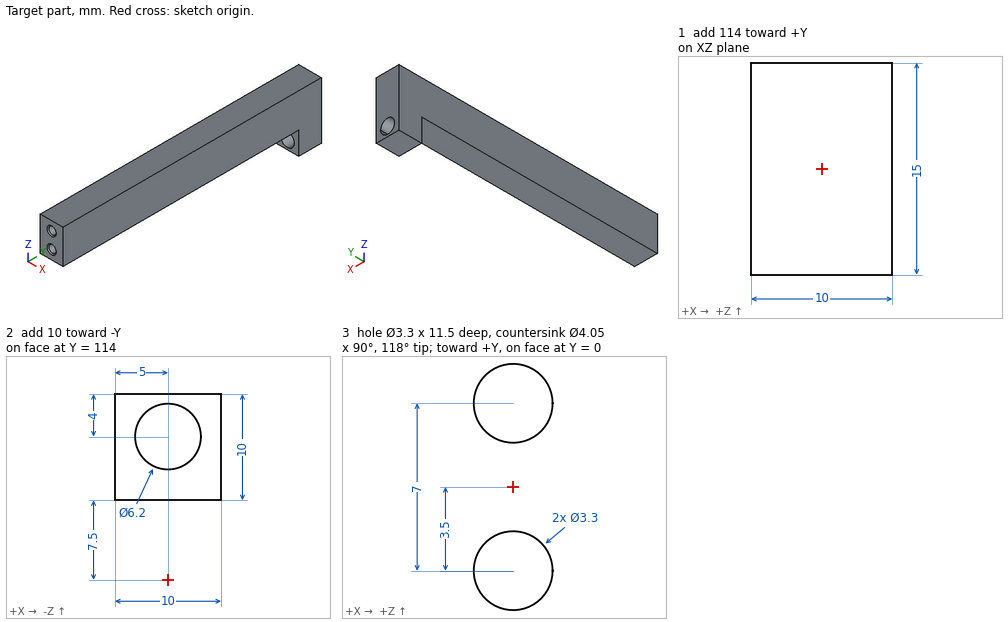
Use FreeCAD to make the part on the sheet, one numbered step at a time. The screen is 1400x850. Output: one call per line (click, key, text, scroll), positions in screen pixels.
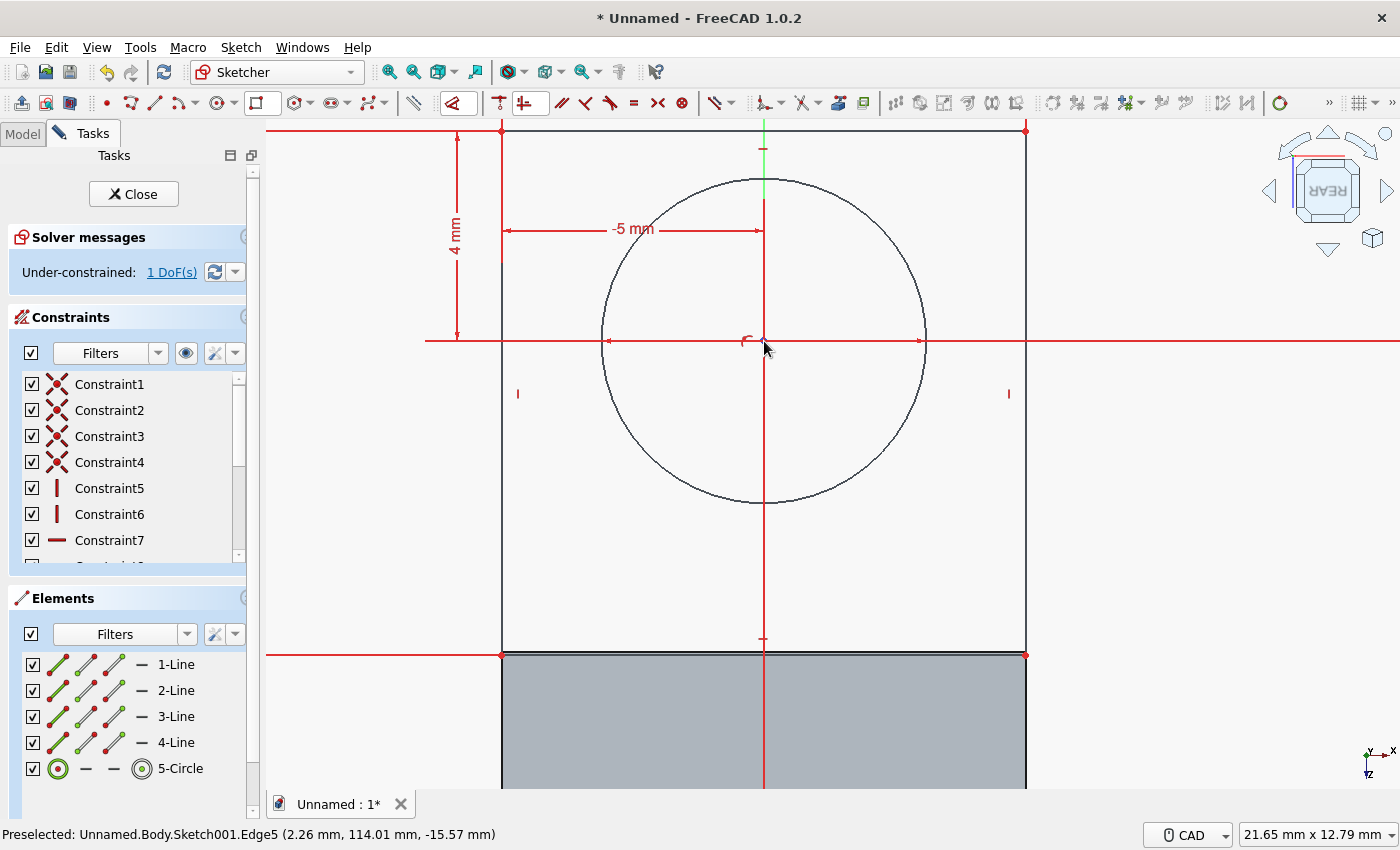
click(502, 655)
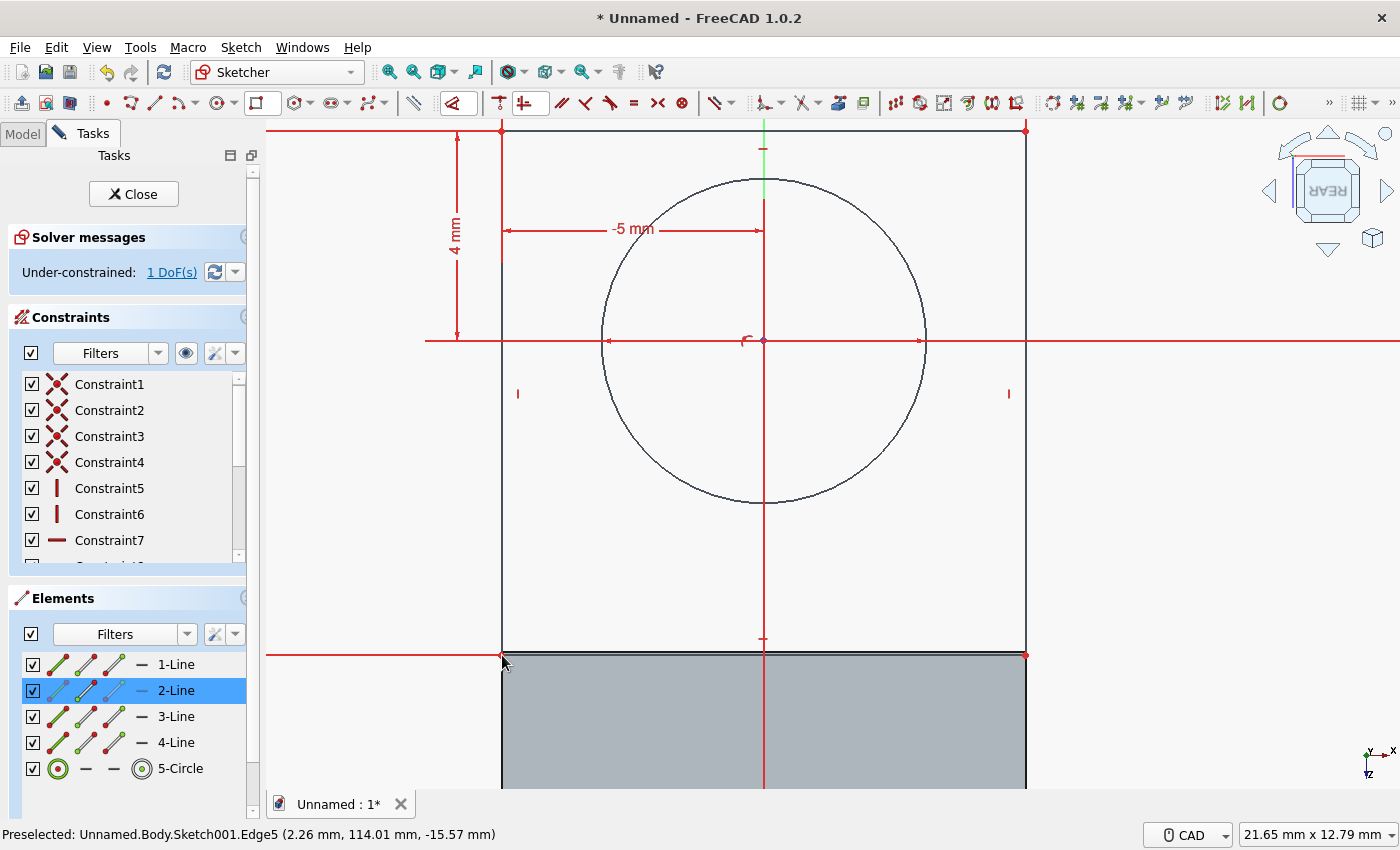
click(472, 104)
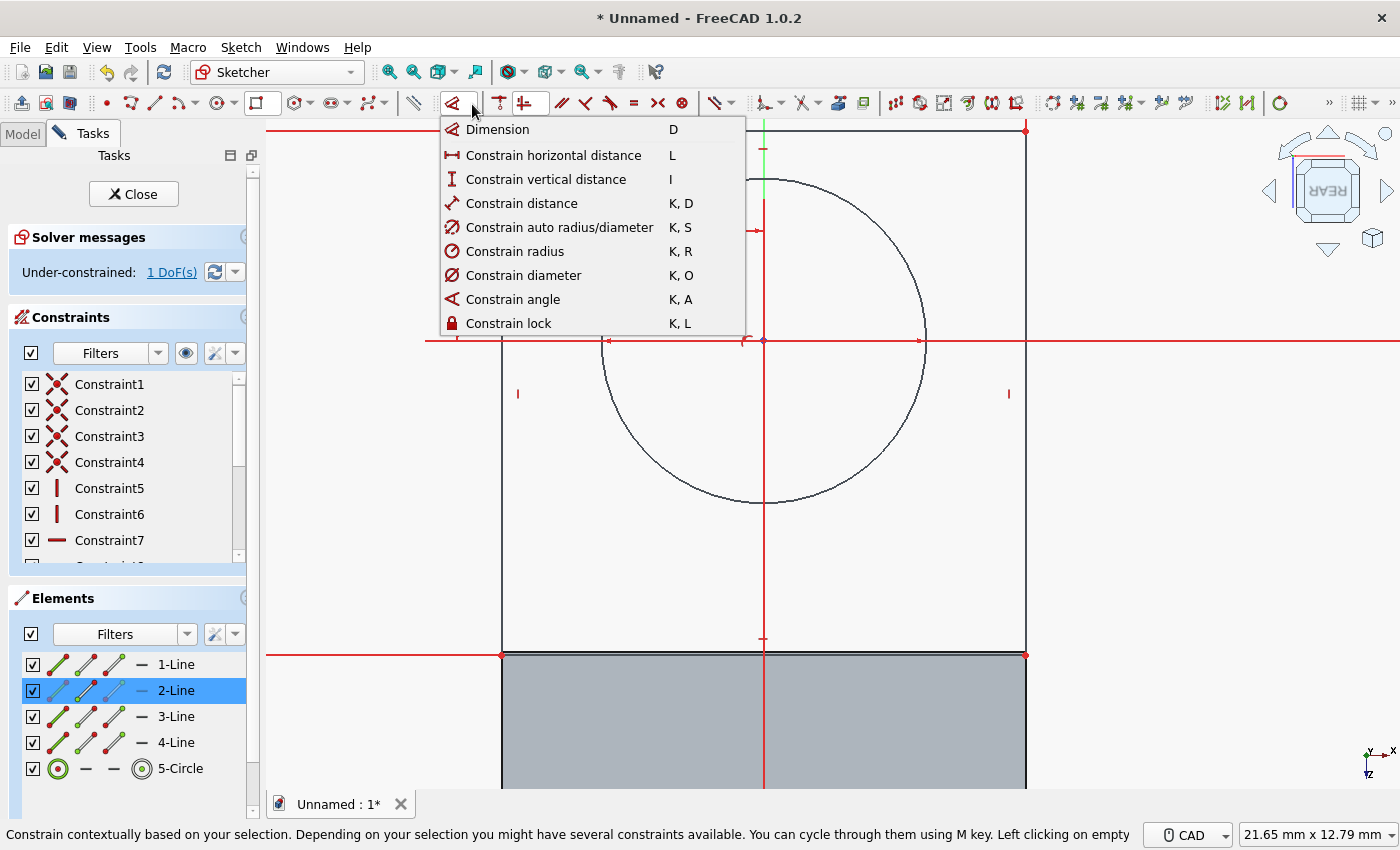
click(593, 179)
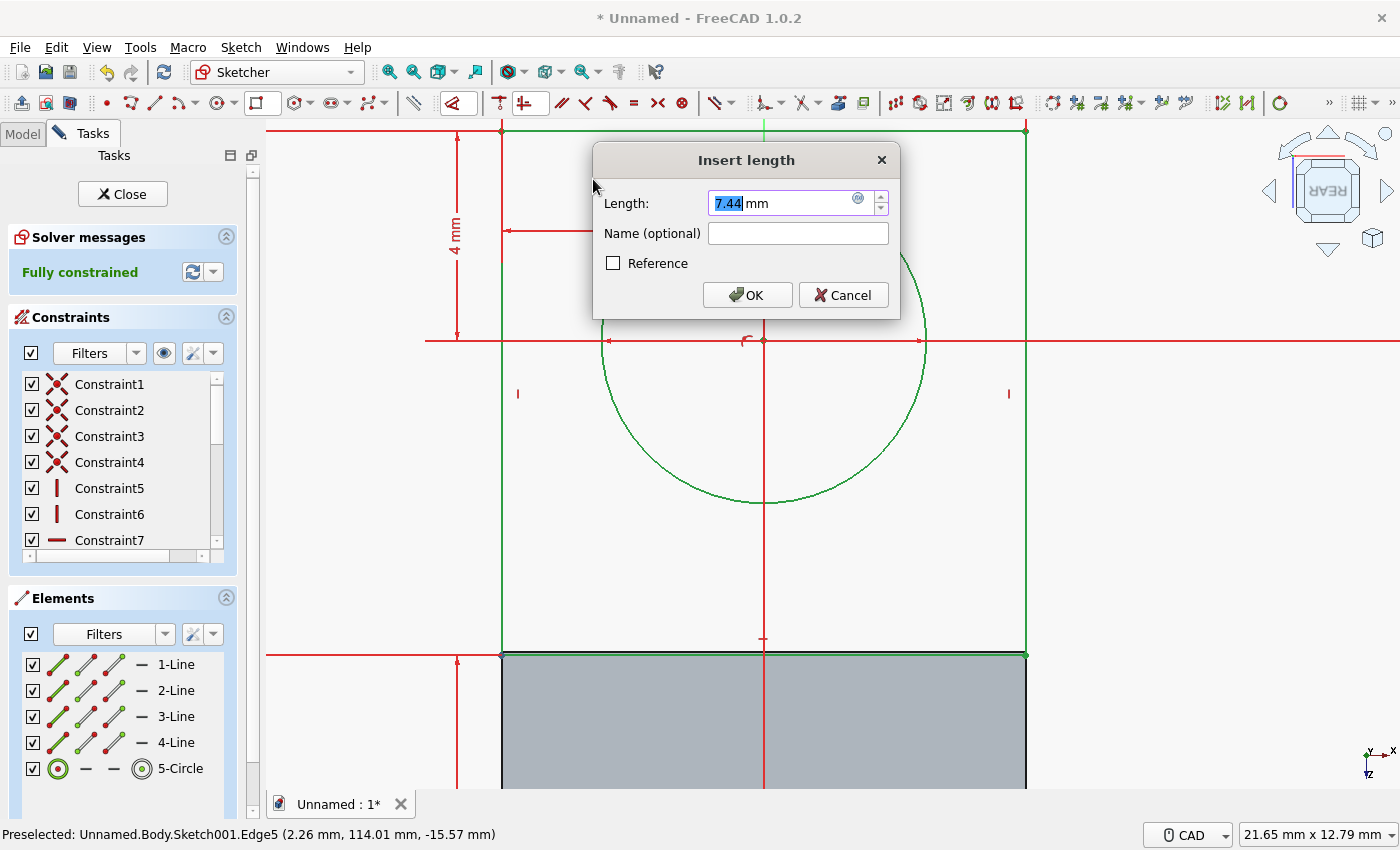
text(7.5)
key(Return)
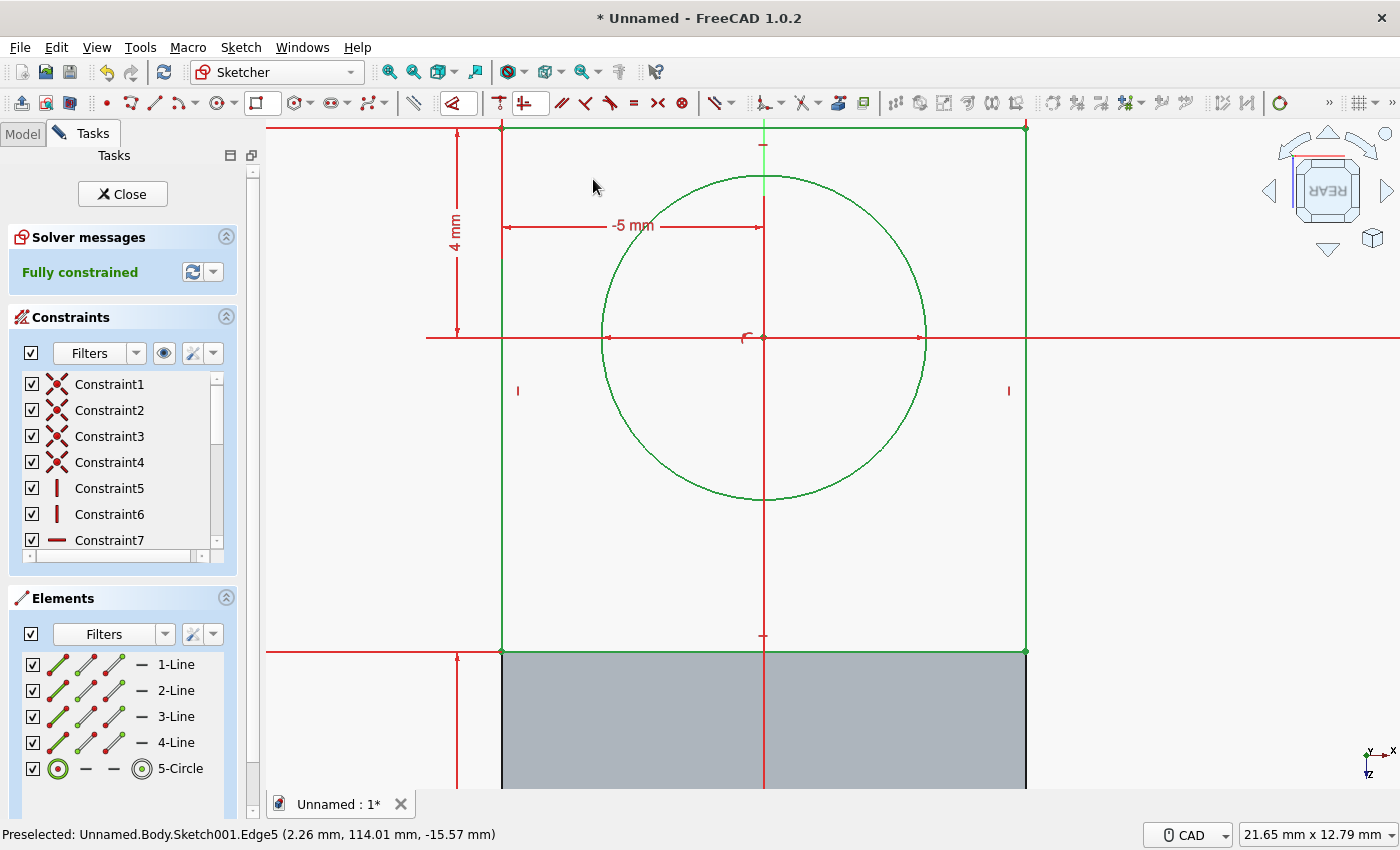
click(123, 194)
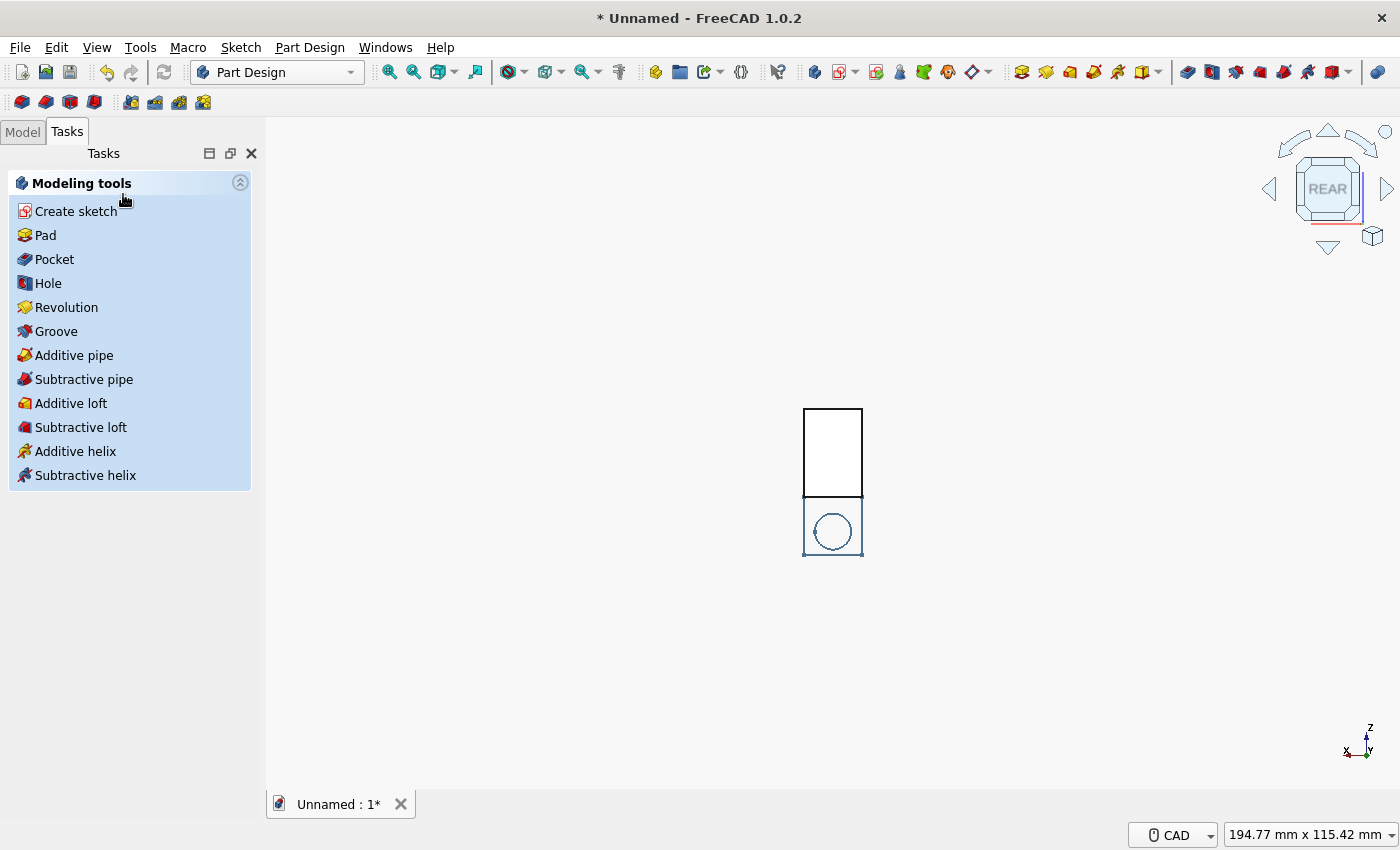
click(1022, 72)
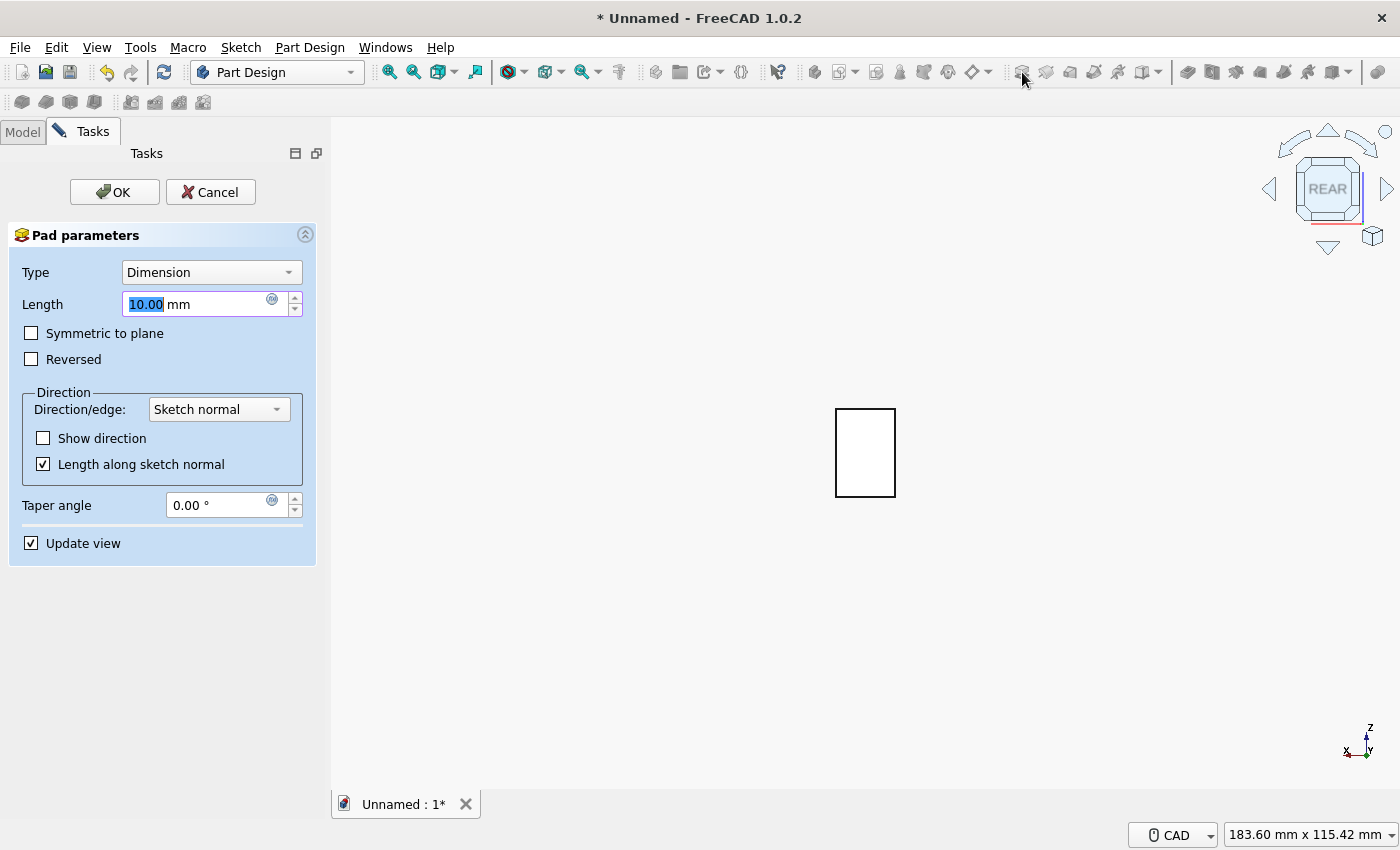
text(10)
key(Tab)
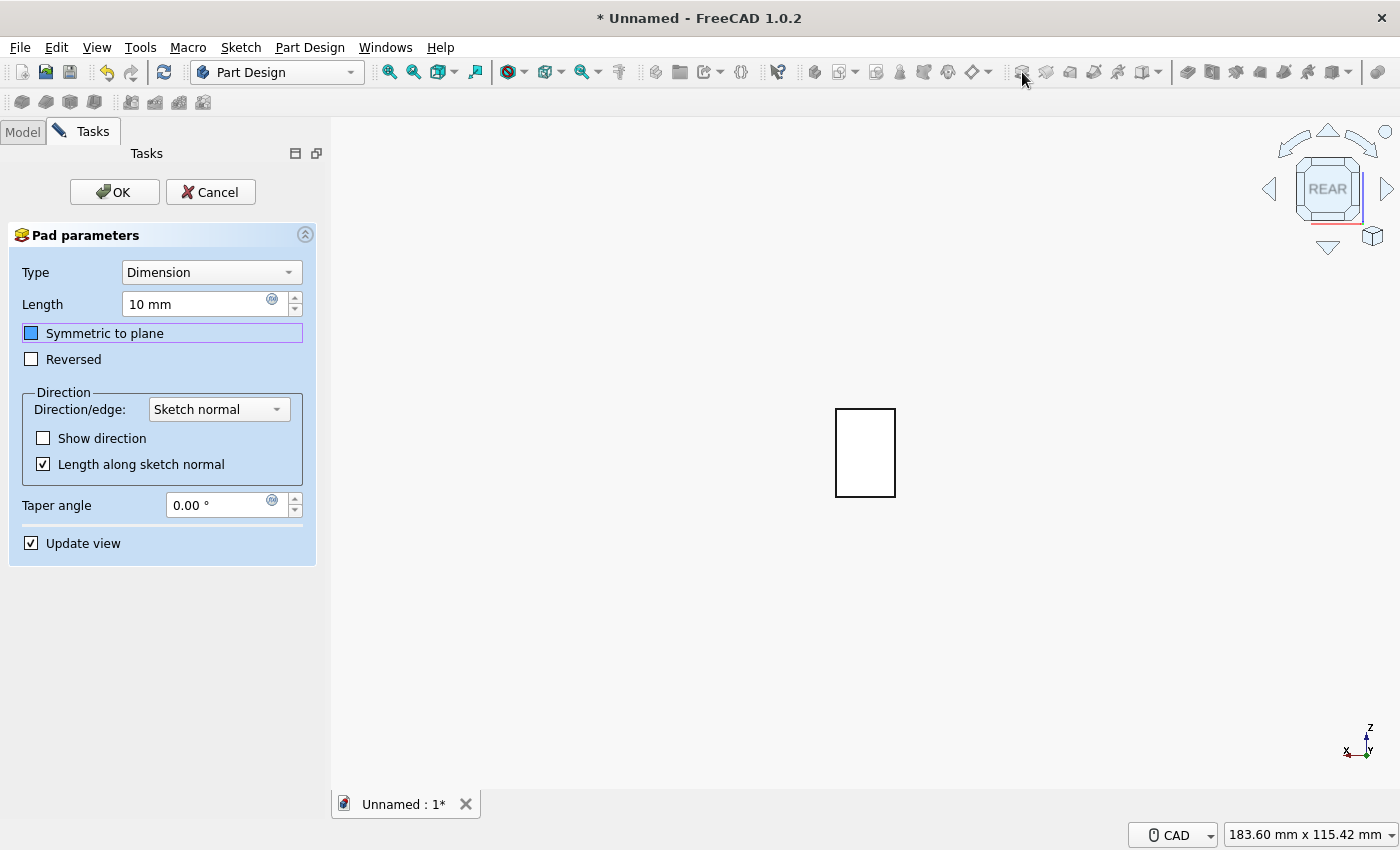
click(30, 359)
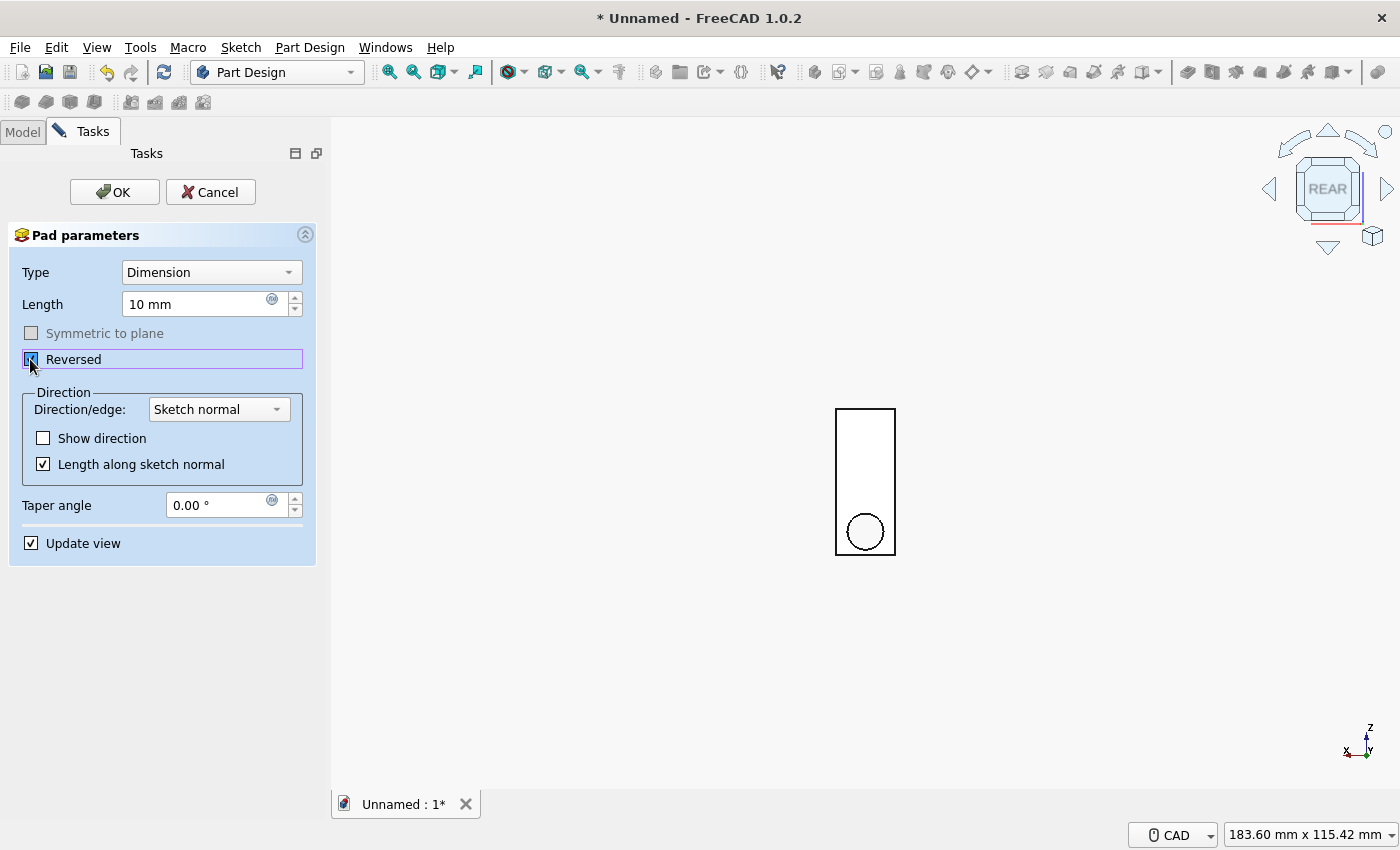
click(115, 192)